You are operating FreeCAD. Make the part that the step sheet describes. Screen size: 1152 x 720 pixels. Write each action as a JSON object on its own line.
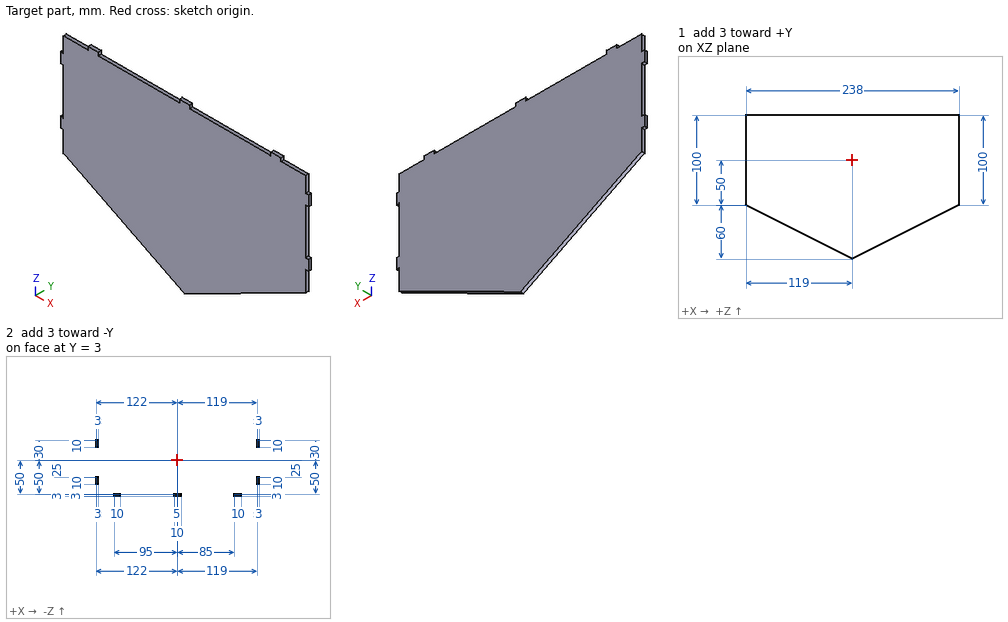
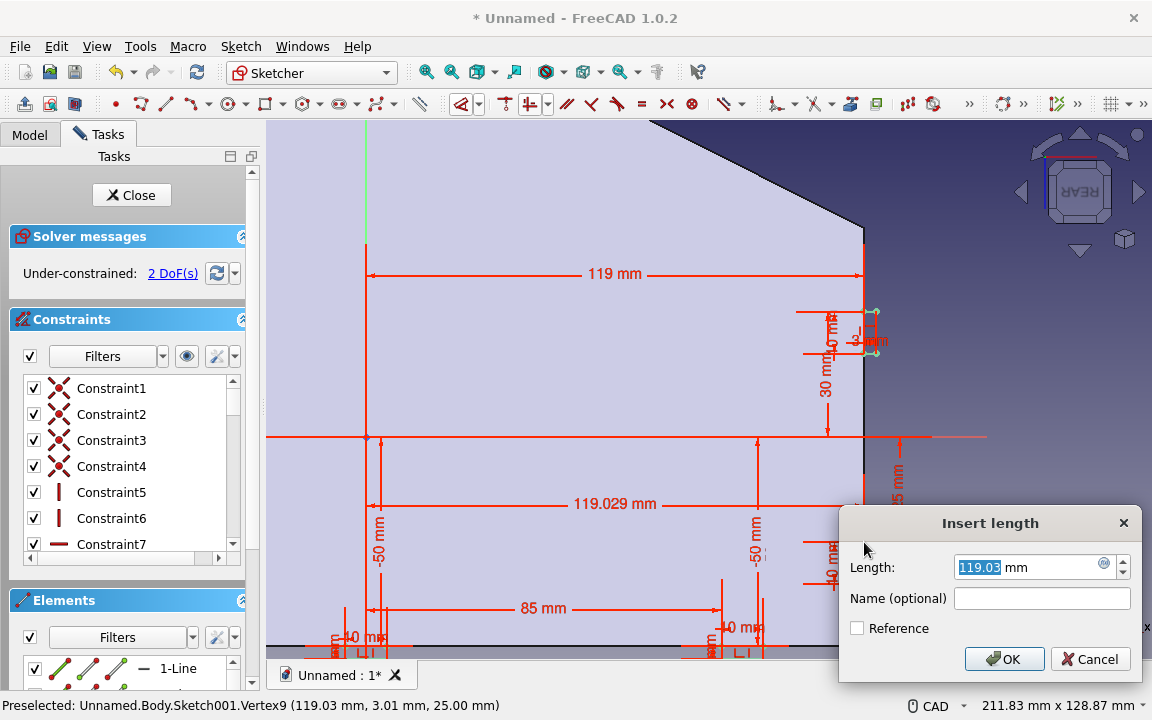
{"action": "type", "text": "119"}
{"action": "key", "text": "Return"}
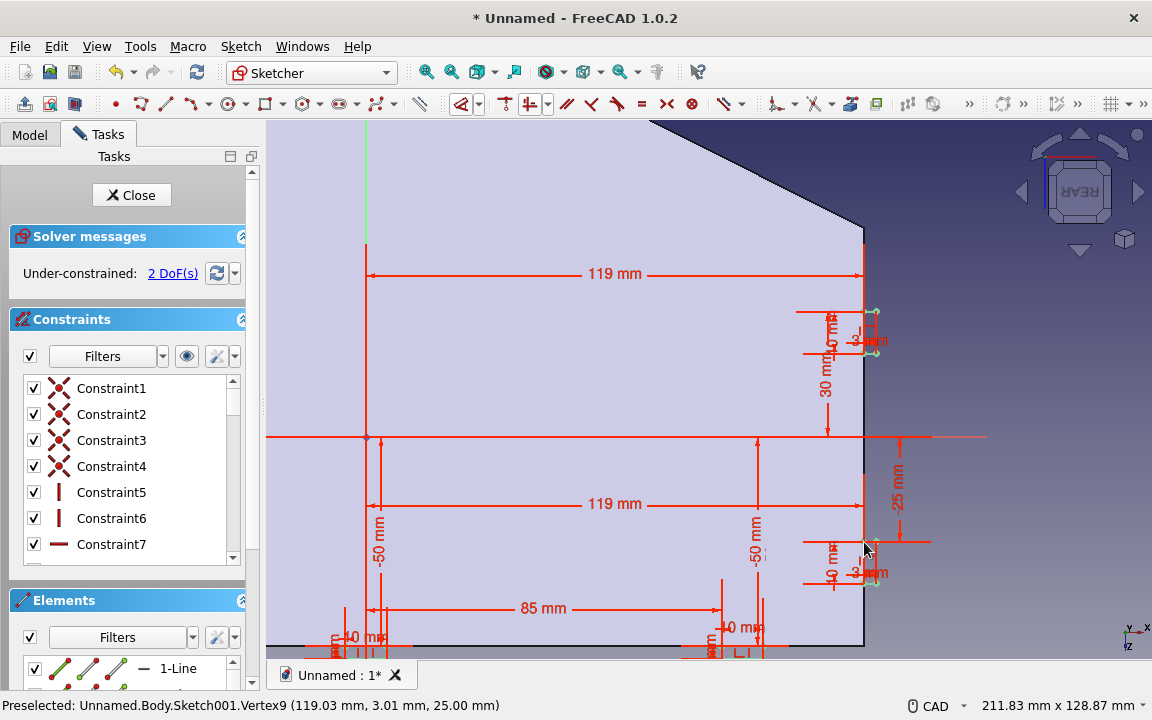
{"action": "scroll", "coordinate": [864, 311], "scroll_direction": "down", "scroll_amount": 4}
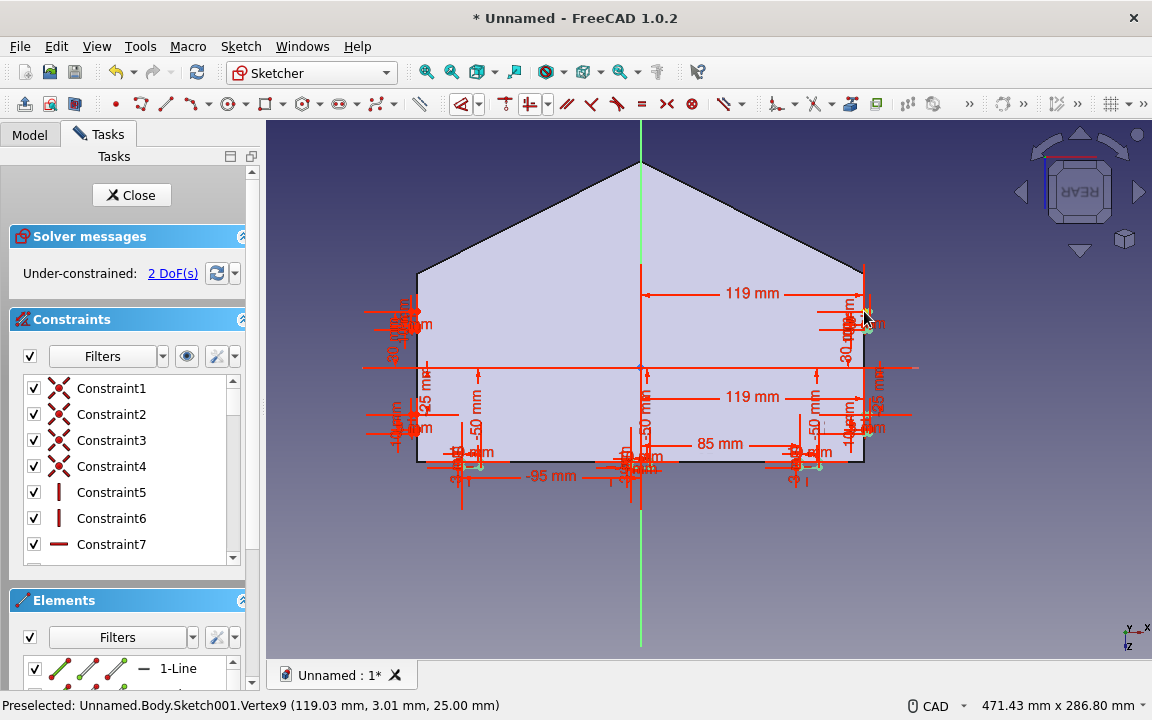
{"action": "scroll", "coordinate": [411, 415], "scroll_direction": "up", "scroll_amount": 4}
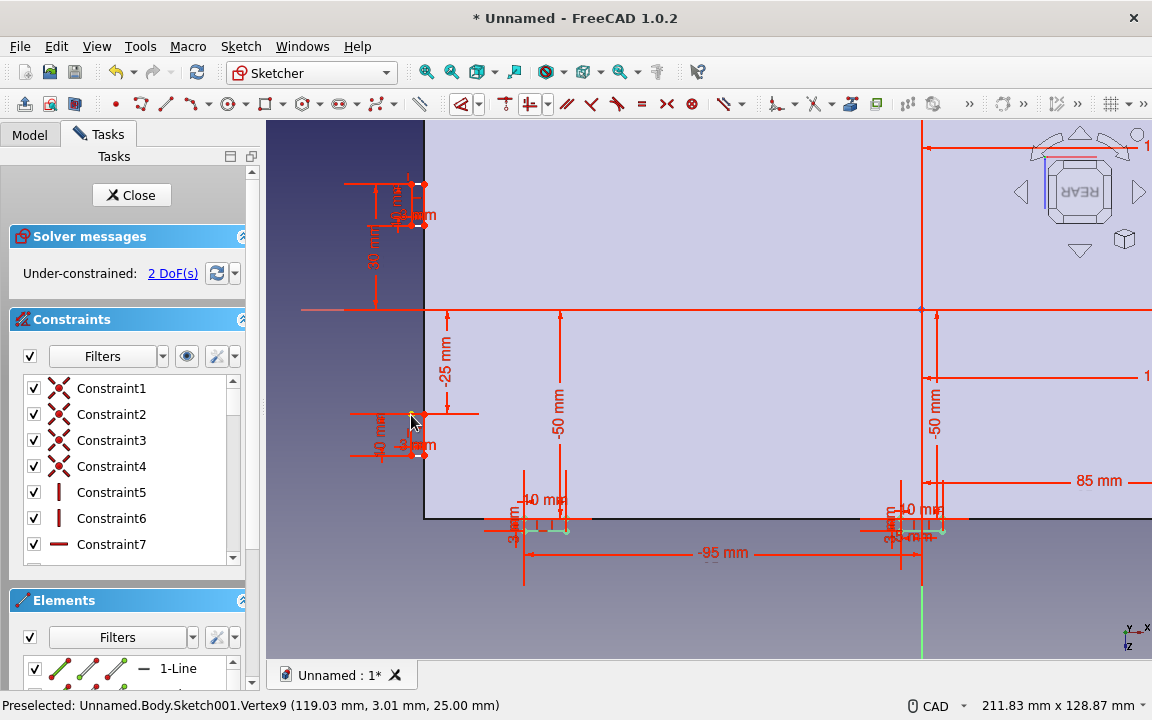
{"action": "left_click", "coordinate": [411, 414]}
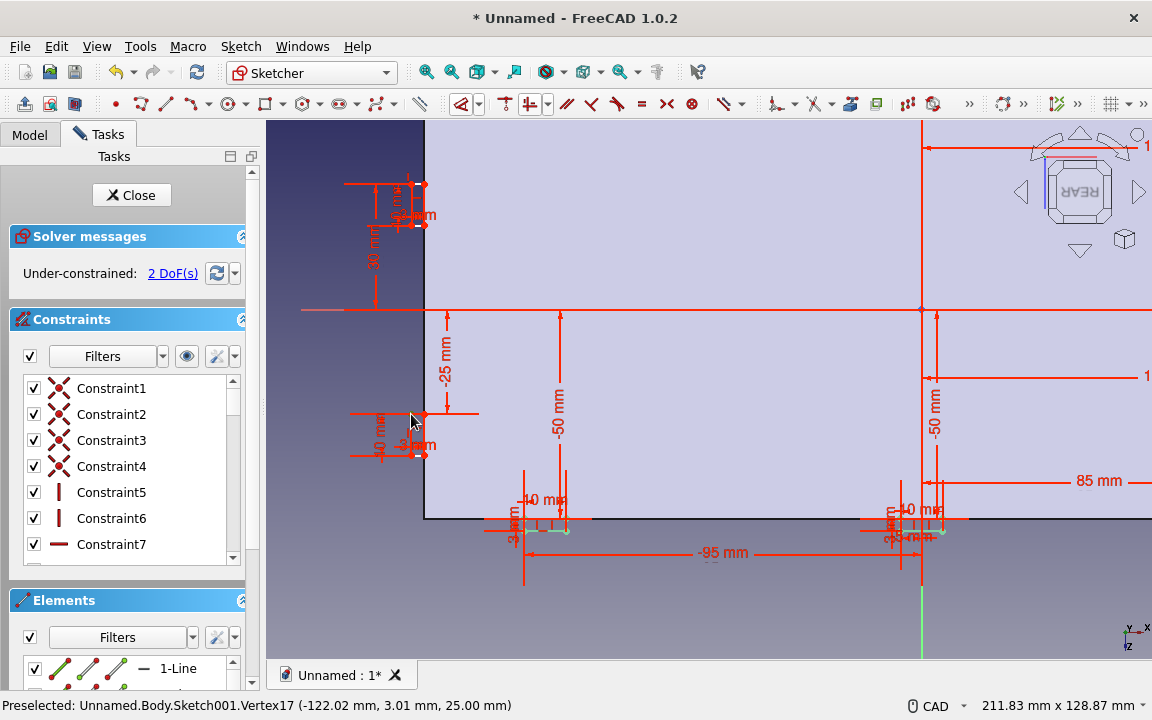
{"action": "key", "text": "l"}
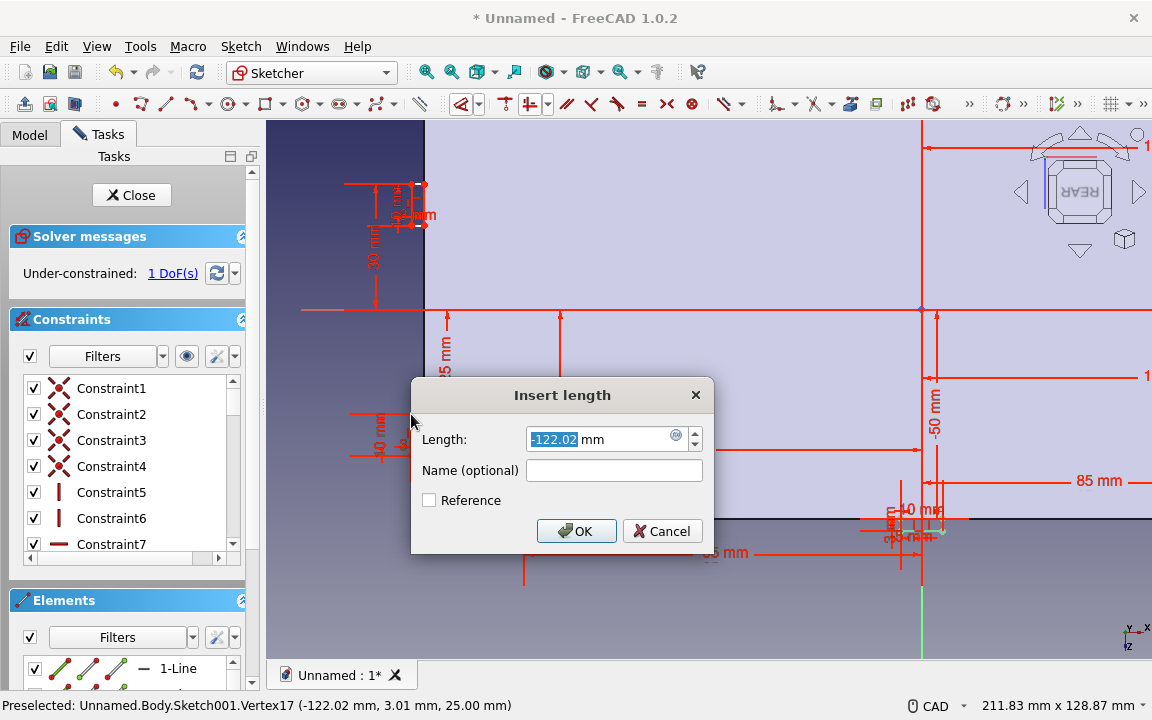
{"action": "type", "text": "-122"}
{"action": "key", "text": "Return"}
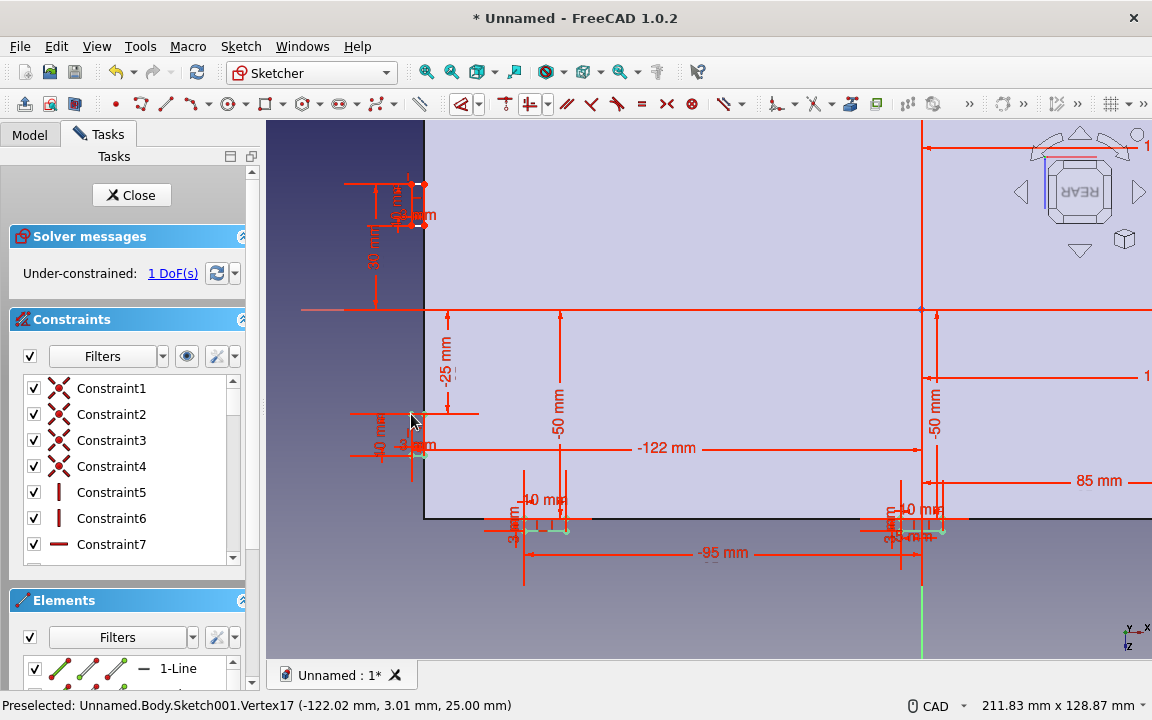
{"action": "left_click", "coordinate": [412, 184]}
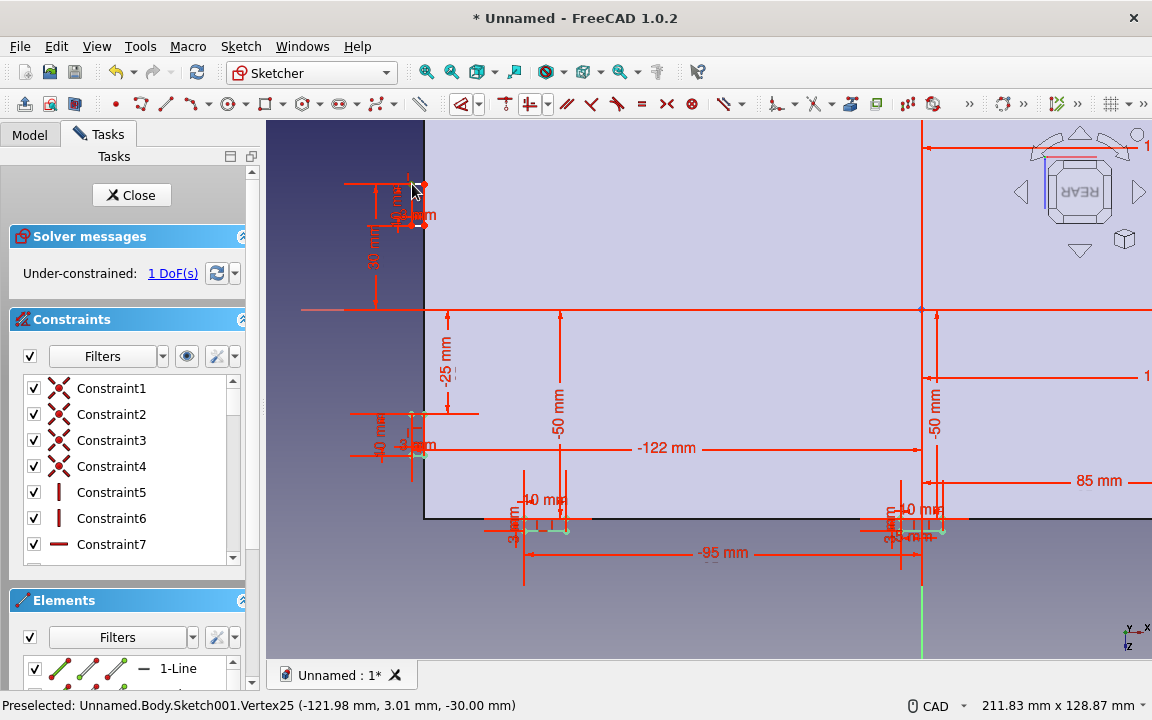
{"action": "key", "text": "l"}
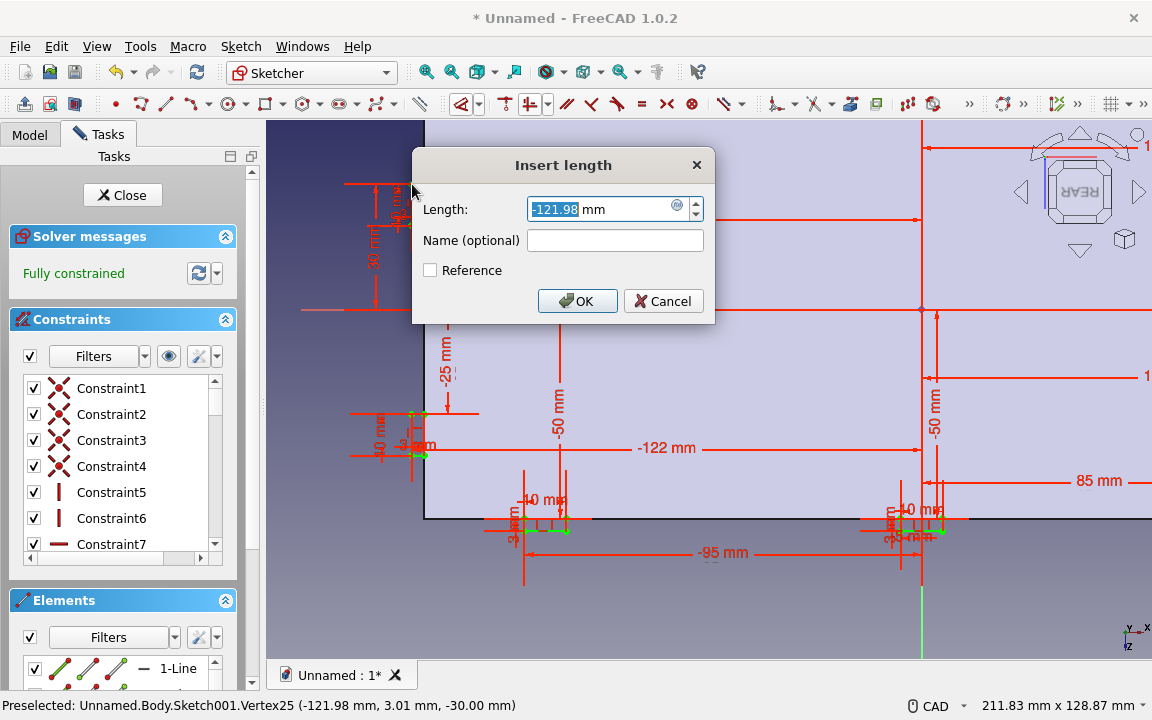
{"action": "type", "text": "-122"}
{"action": "key", "text": "Return"}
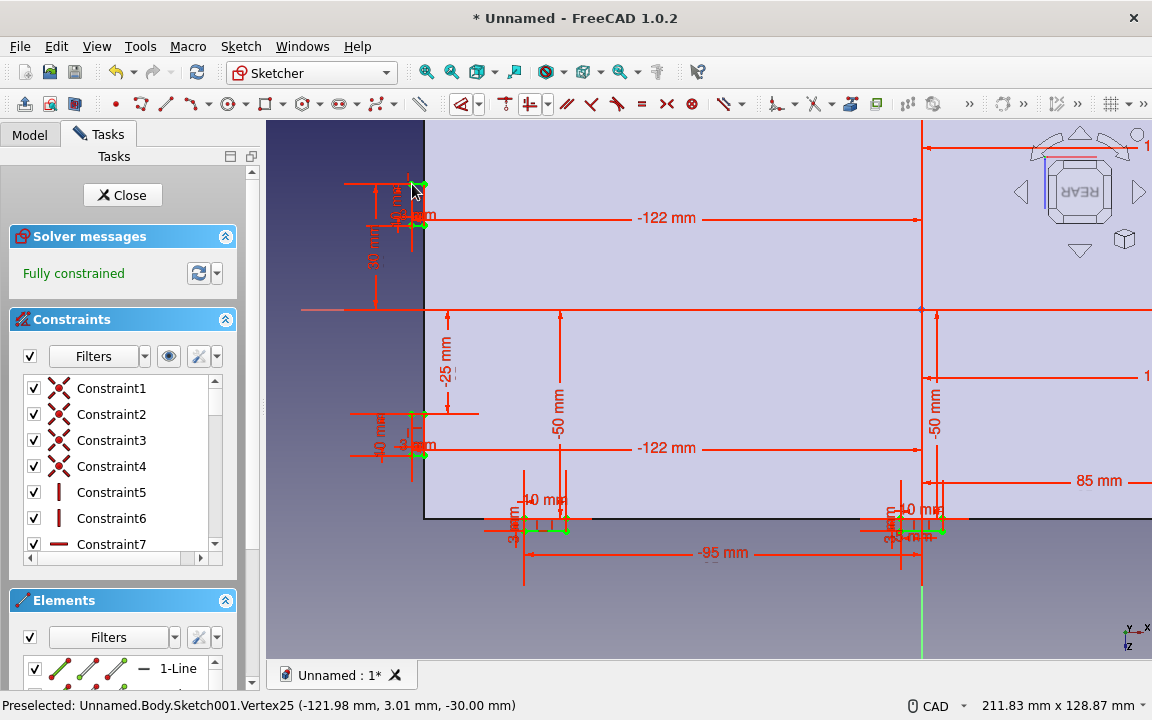
{"action": "left_click", "coordinate": [123, 195]}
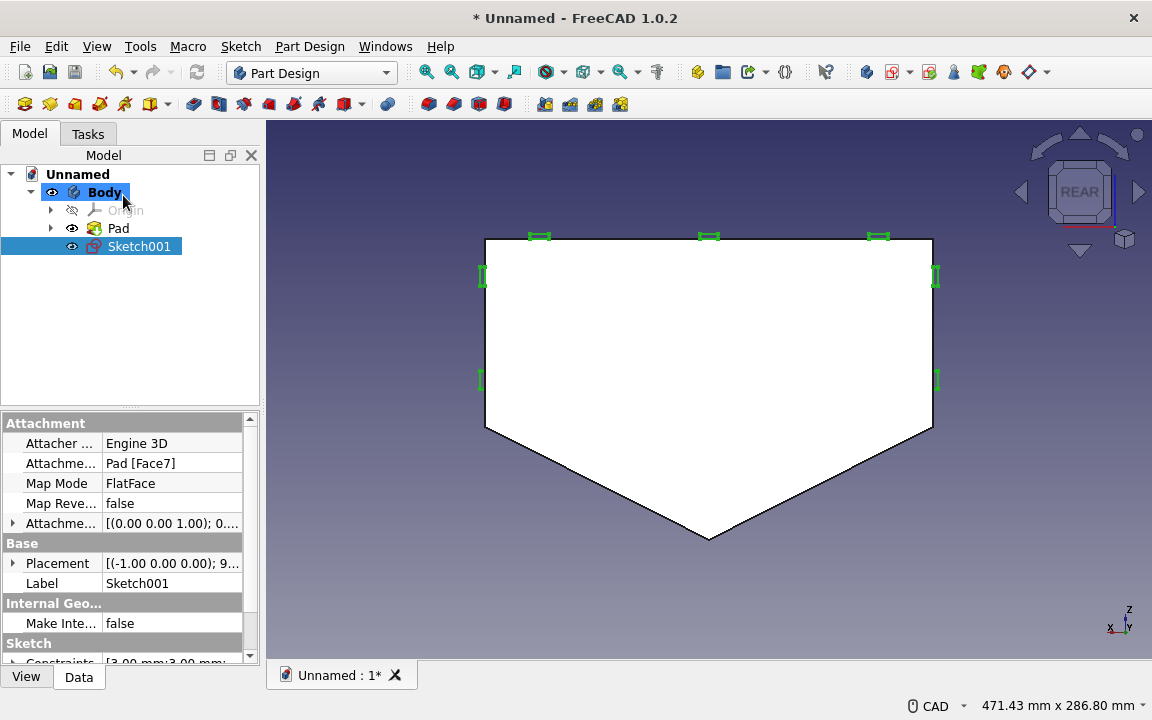
{"action": "left_click", "coordinate": [25, 104]}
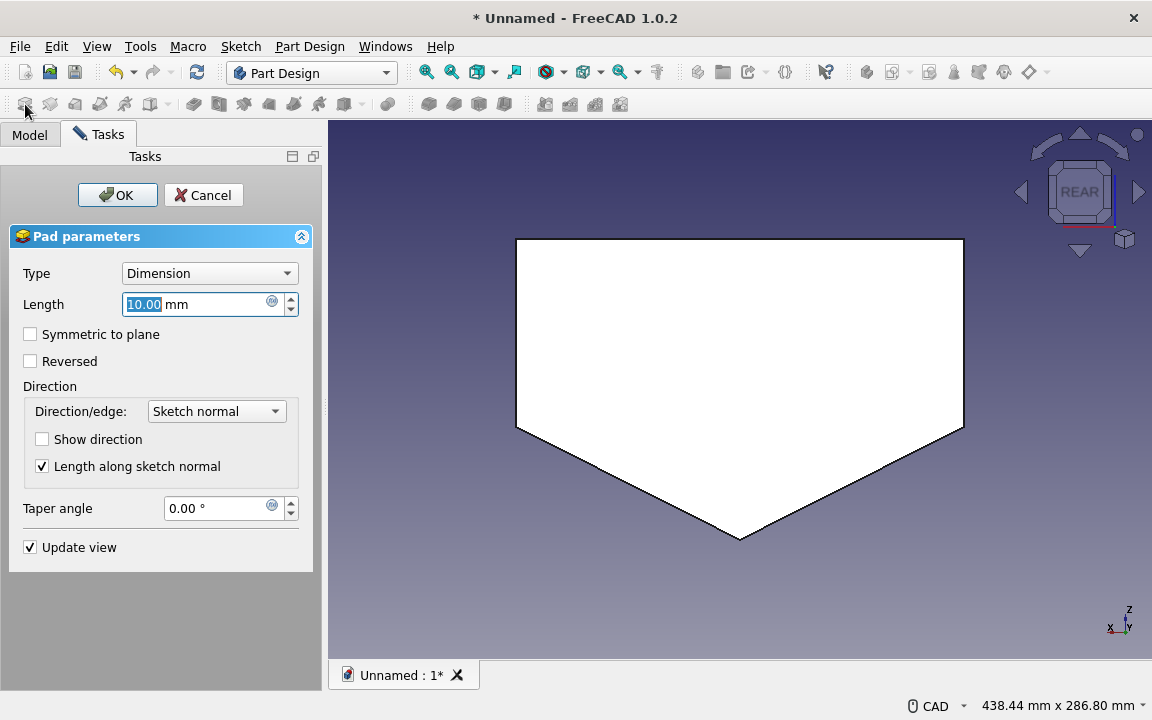
{"action": "type", "text": "3"}
{"action": "key", "text": "Tab"}